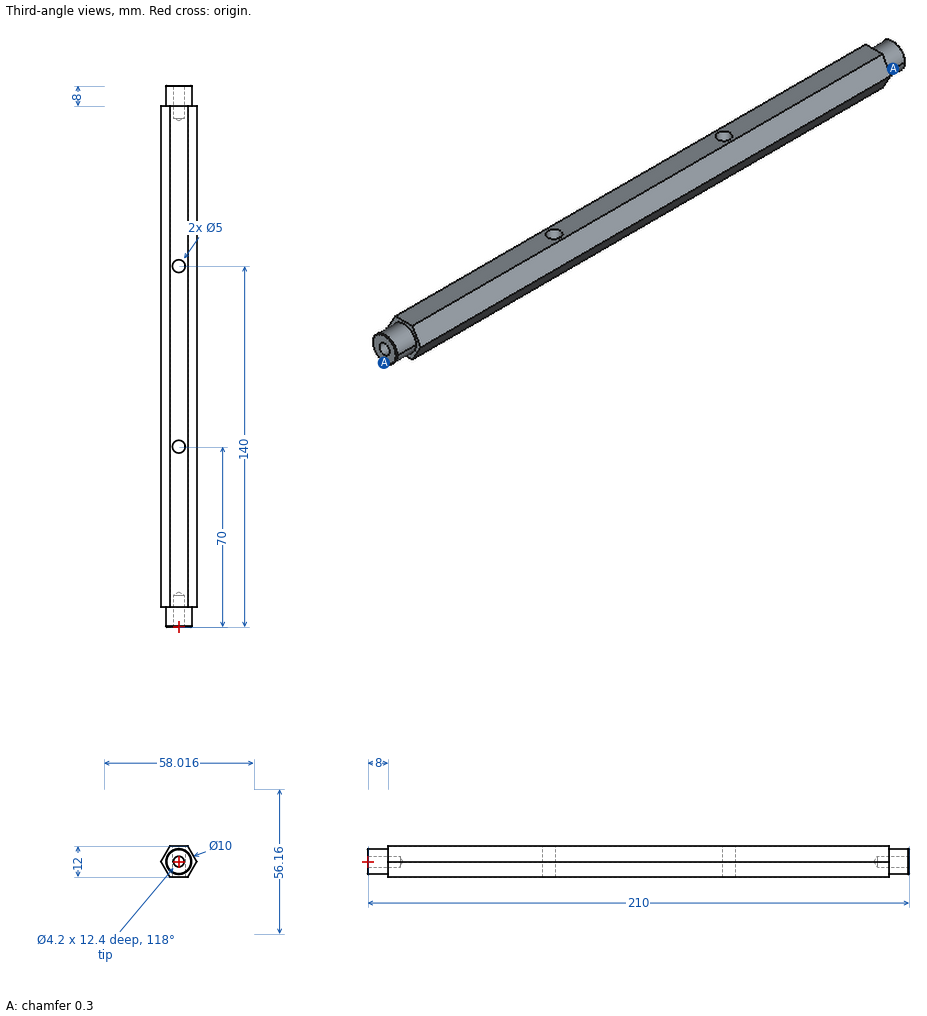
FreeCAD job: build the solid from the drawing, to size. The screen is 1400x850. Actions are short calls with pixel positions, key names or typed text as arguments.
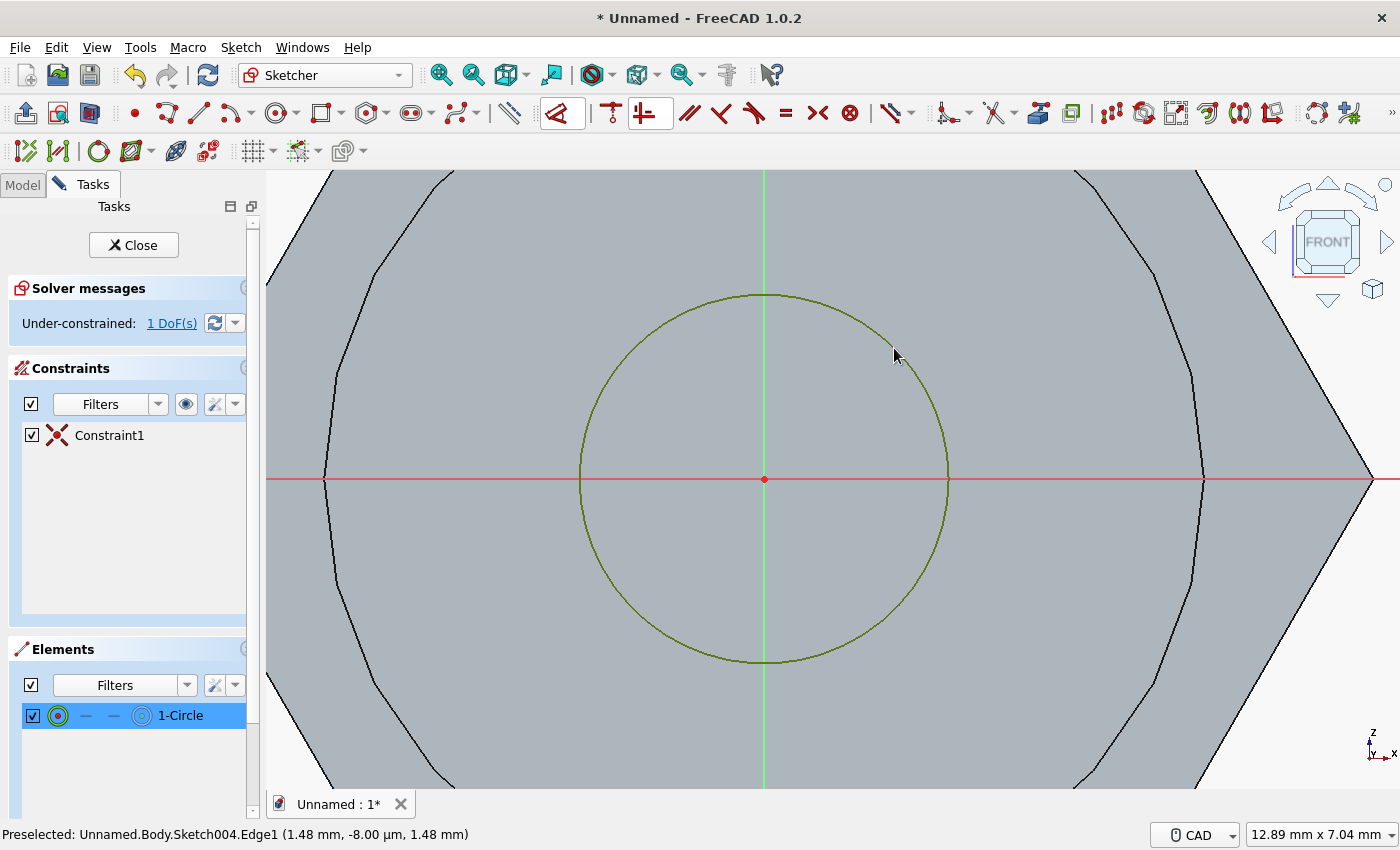
click(580, 114)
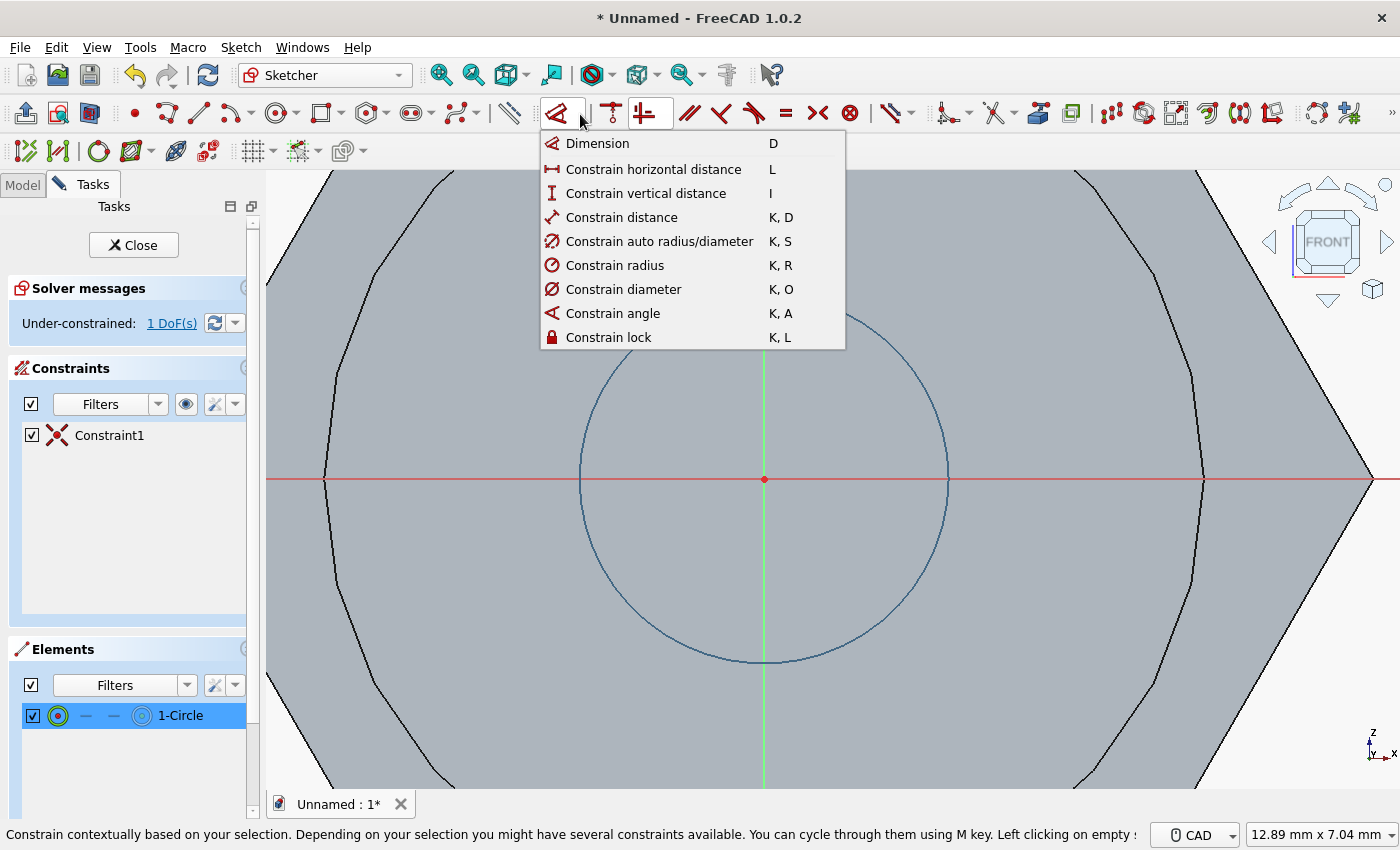
click(693, 289)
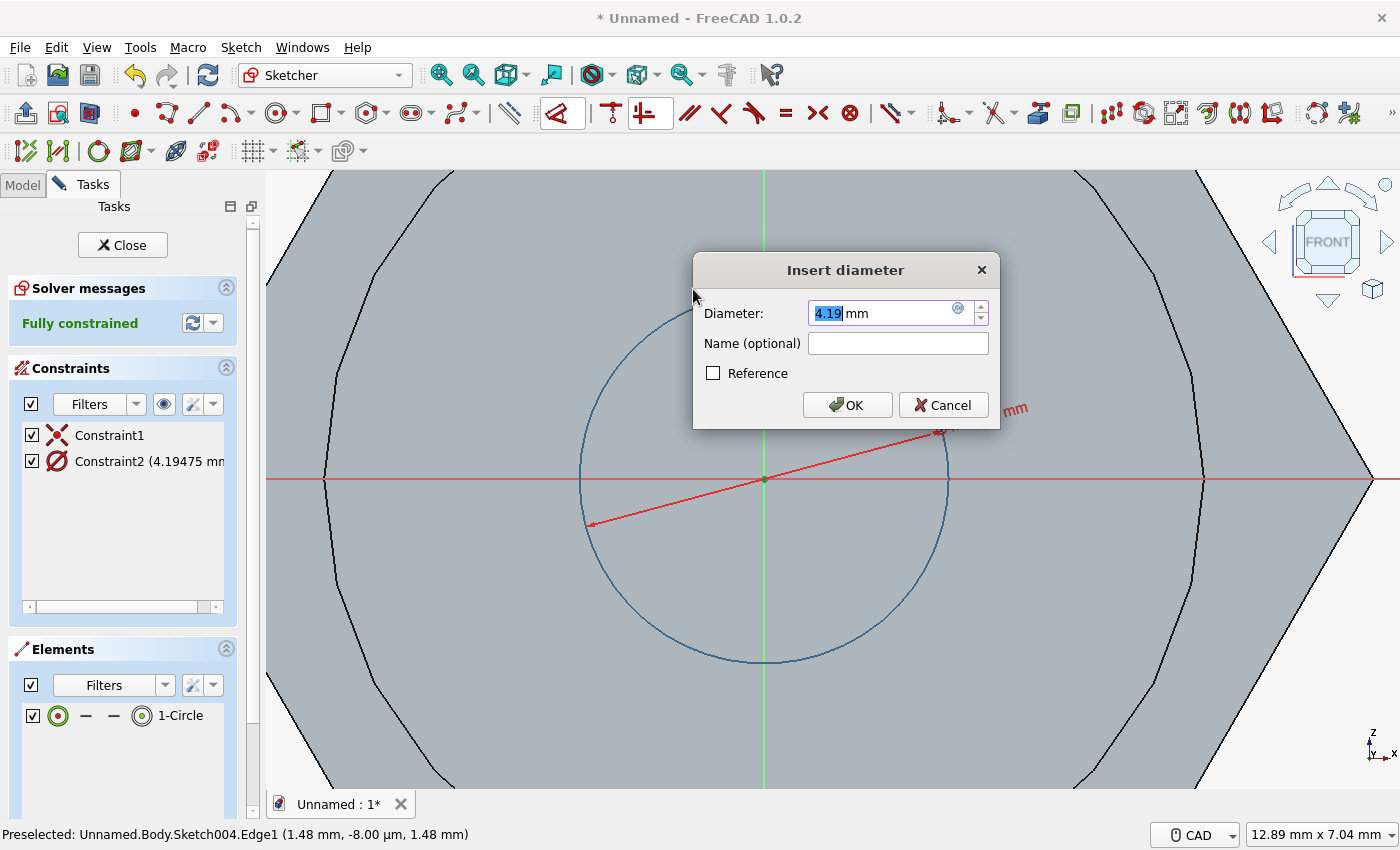
text(4.2)
key(Return)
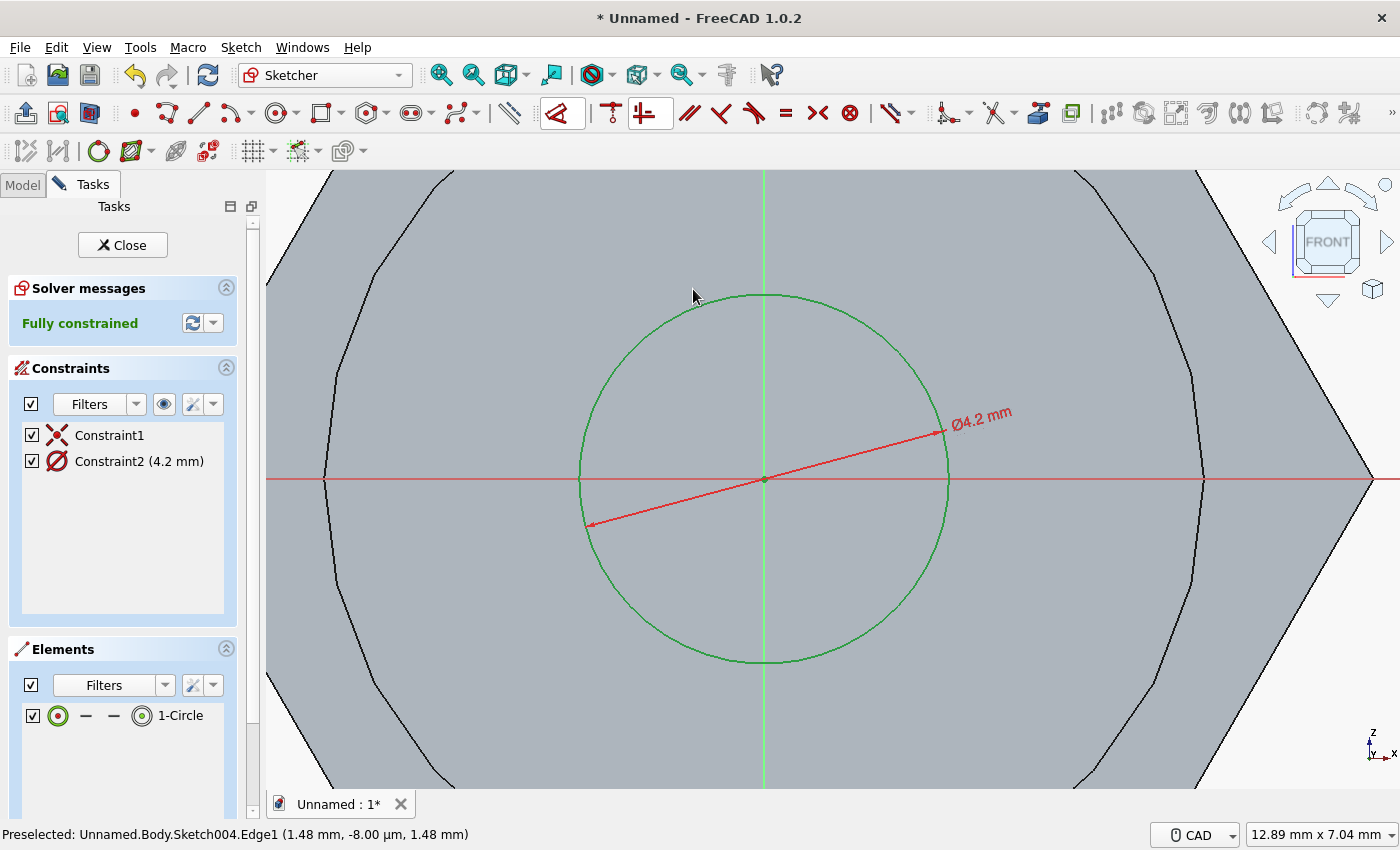
click(123, 245)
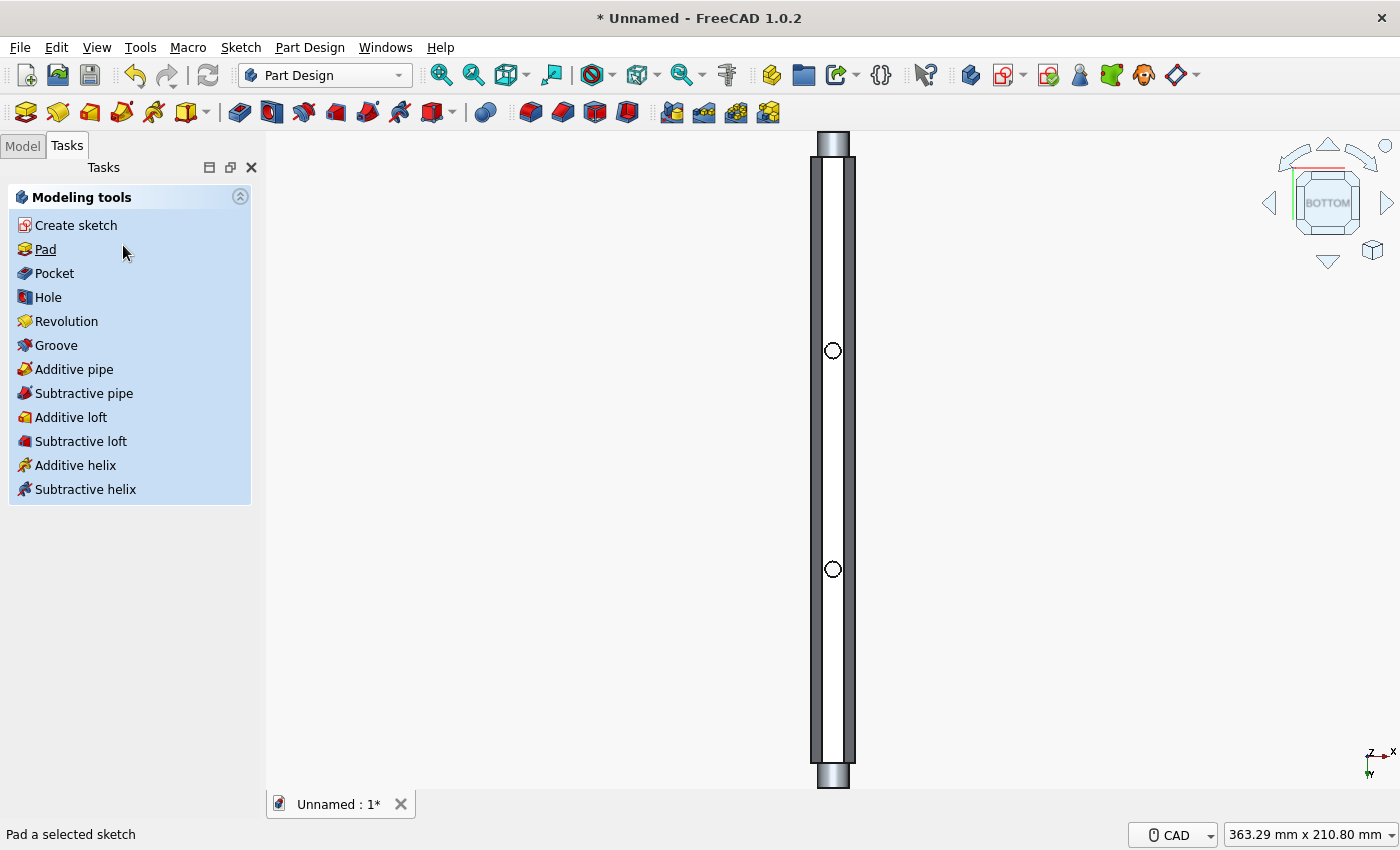
click(272, 112)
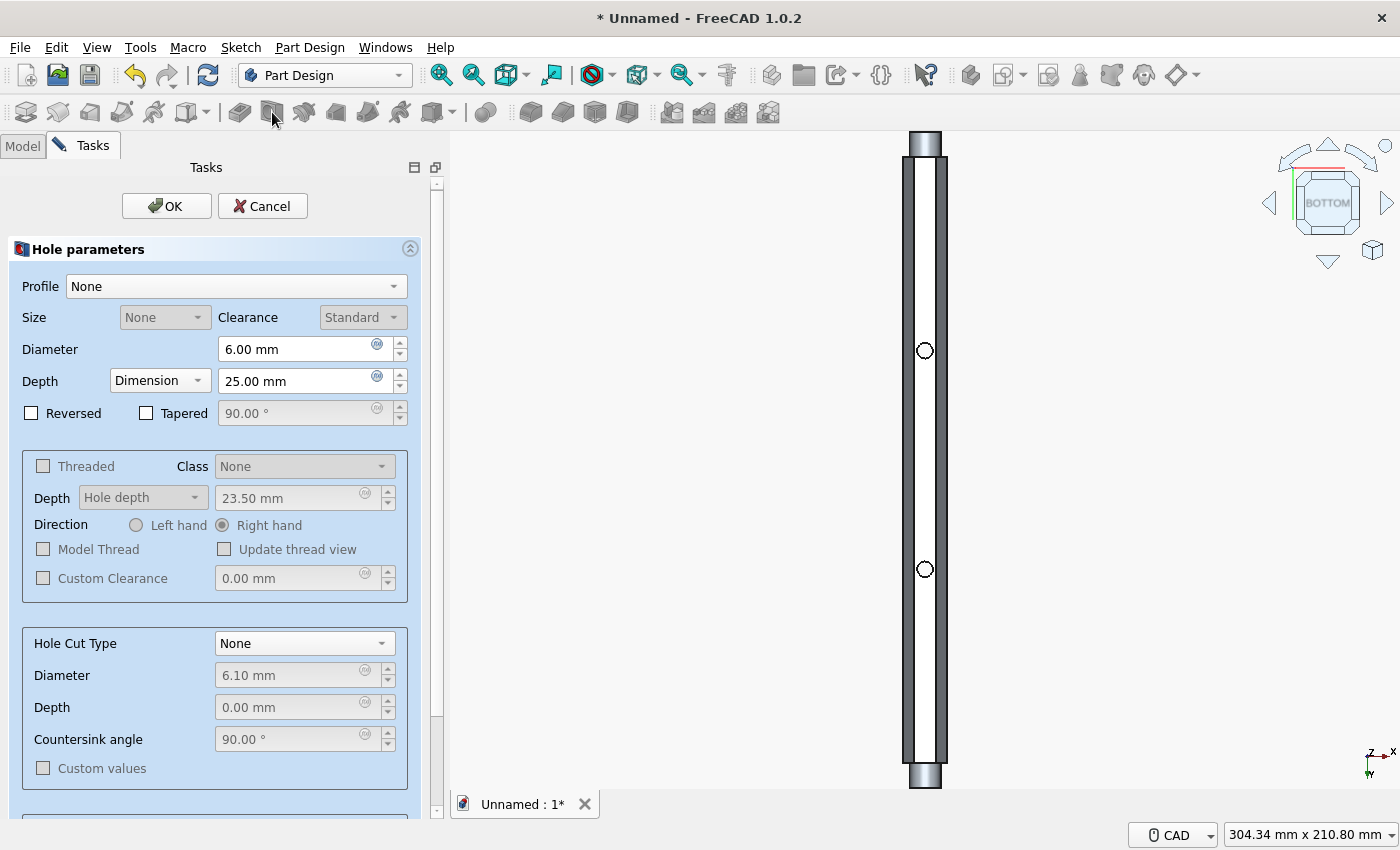
triple_click(305, 349)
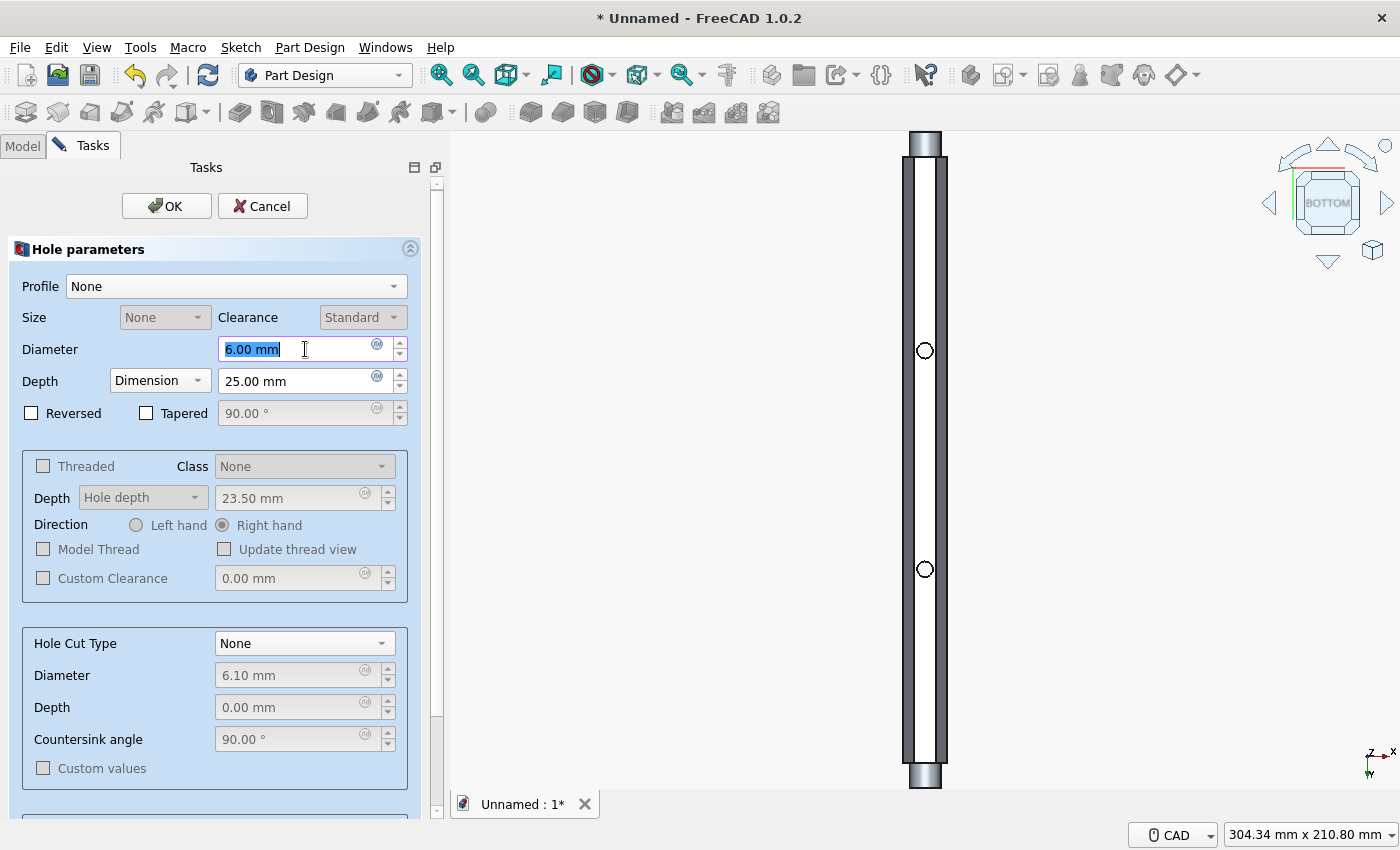
text(4.2)
key(Tab)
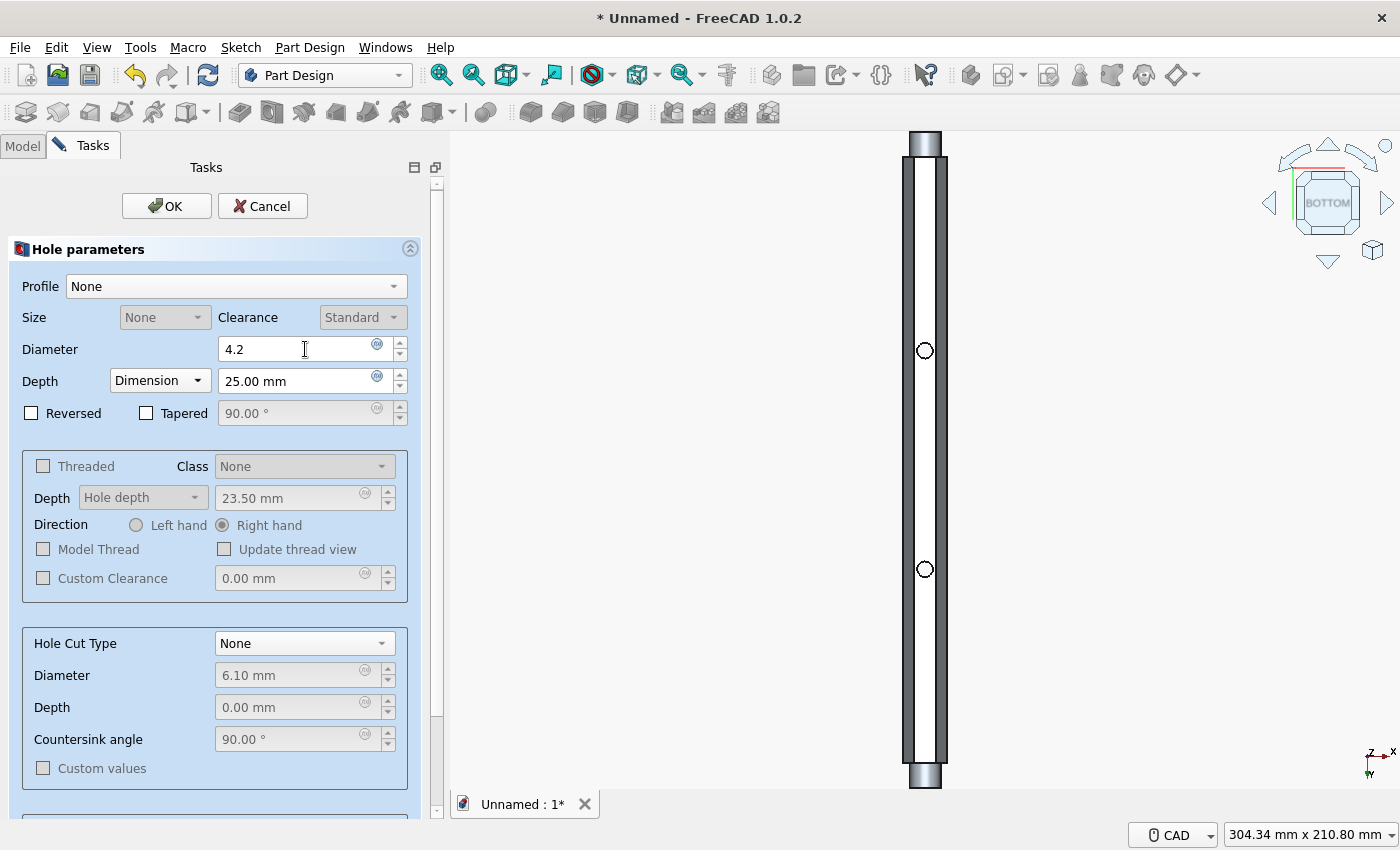
triple_click(305, 381)